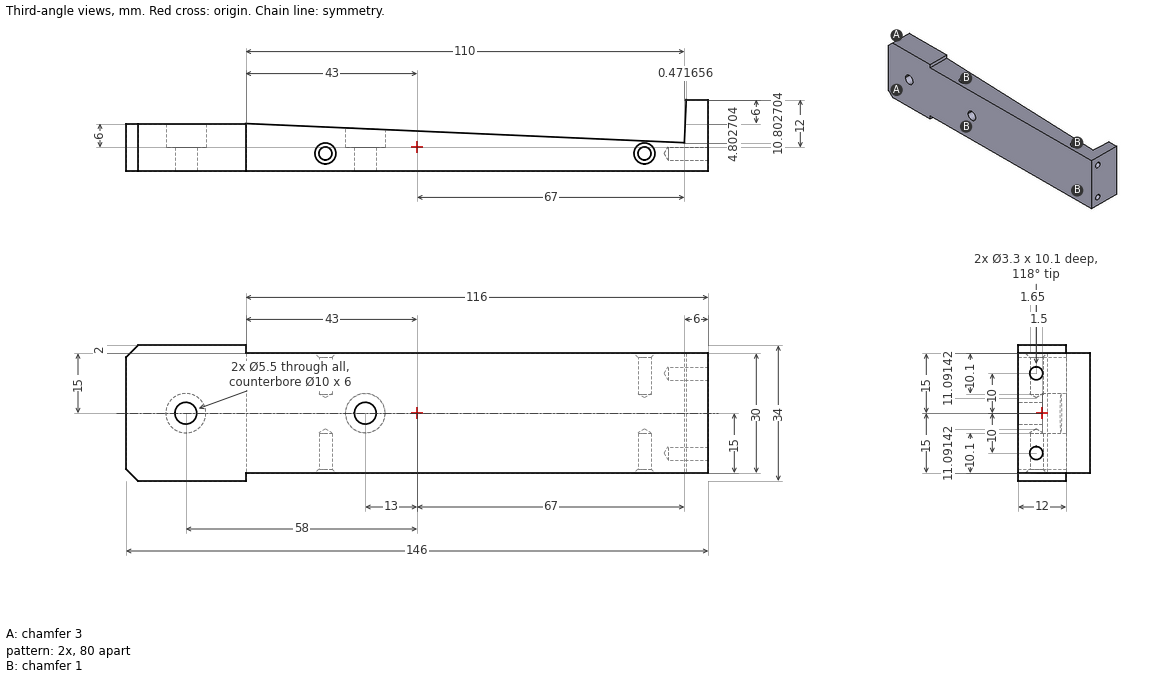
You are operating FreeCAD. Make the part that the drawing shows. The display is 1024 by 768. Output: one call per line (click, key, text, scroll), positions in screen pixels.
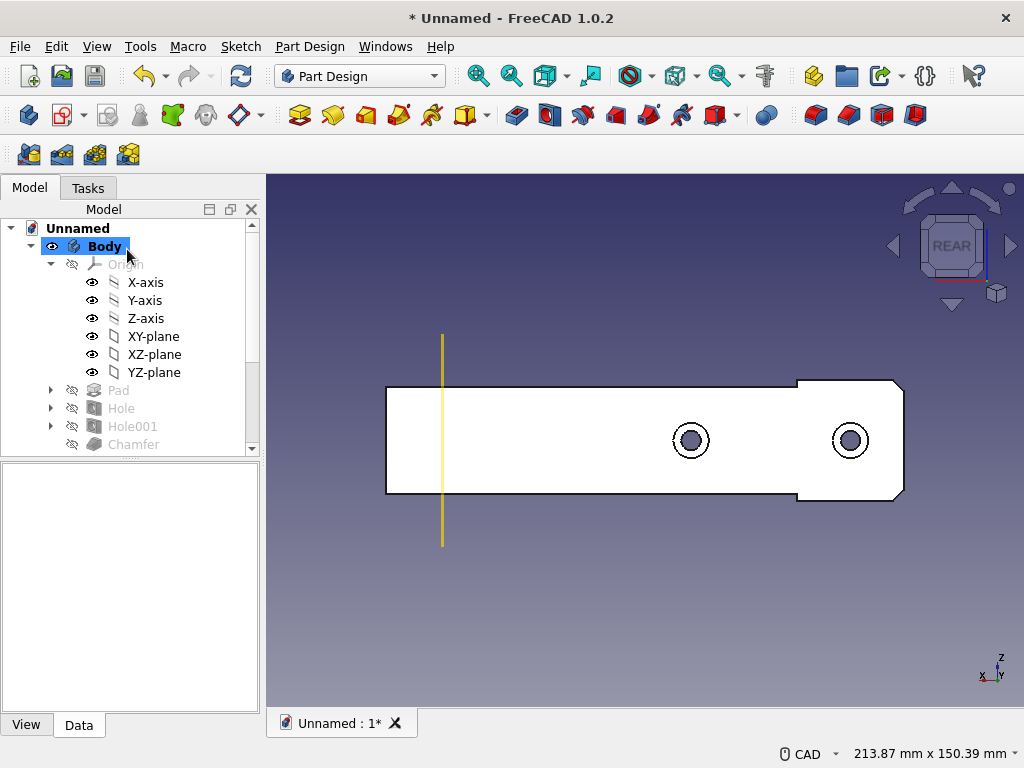
scroll(101, 332, down, 3)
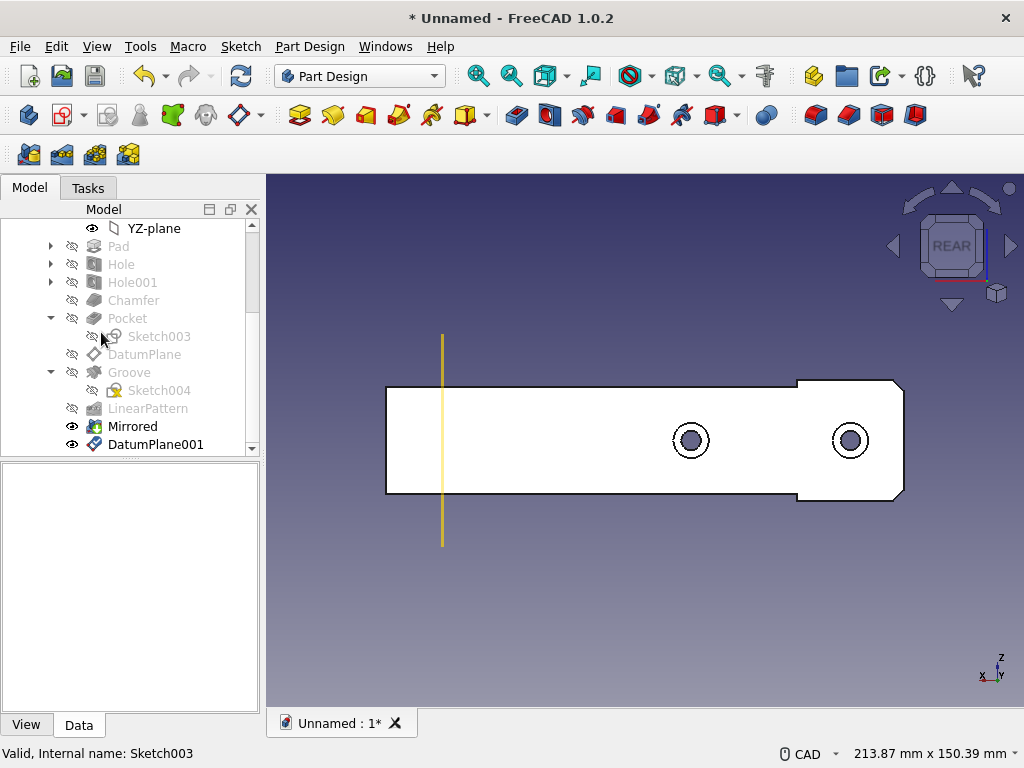
click(117, 444)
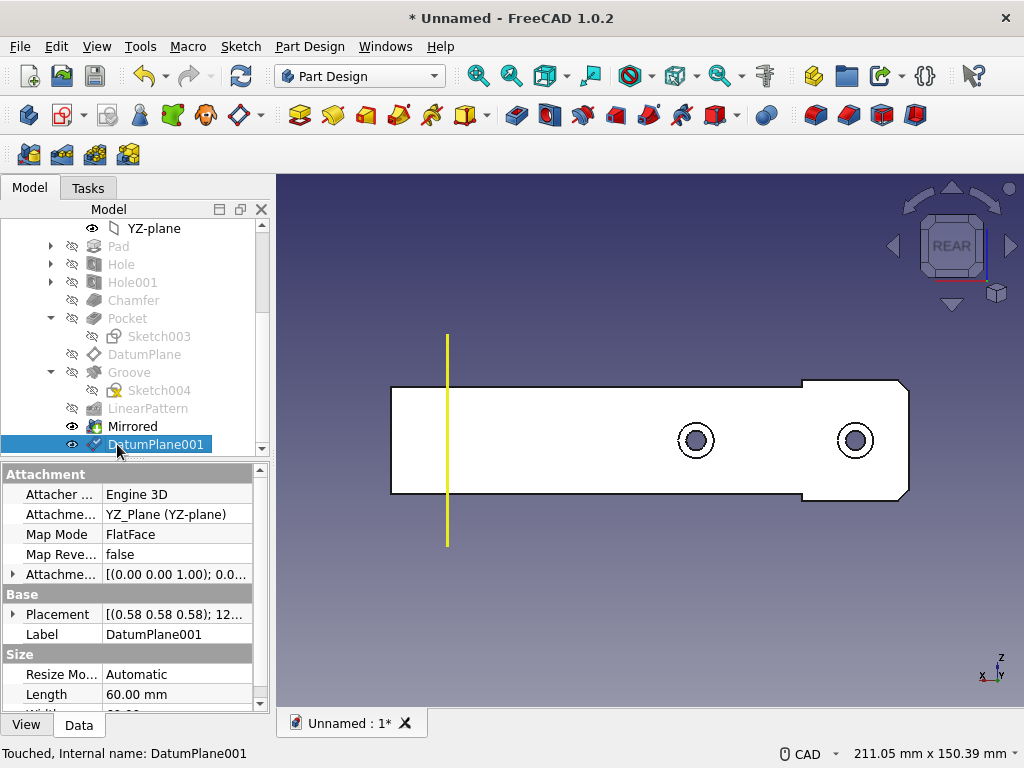
click(62, 116)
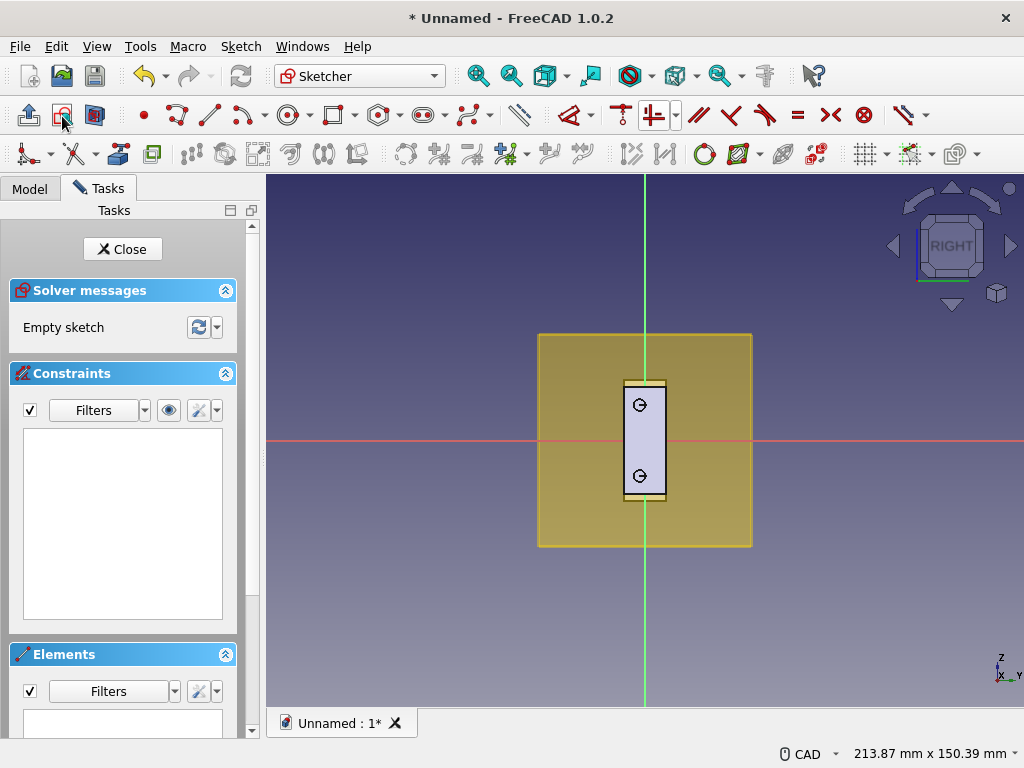
key(q)
key(s)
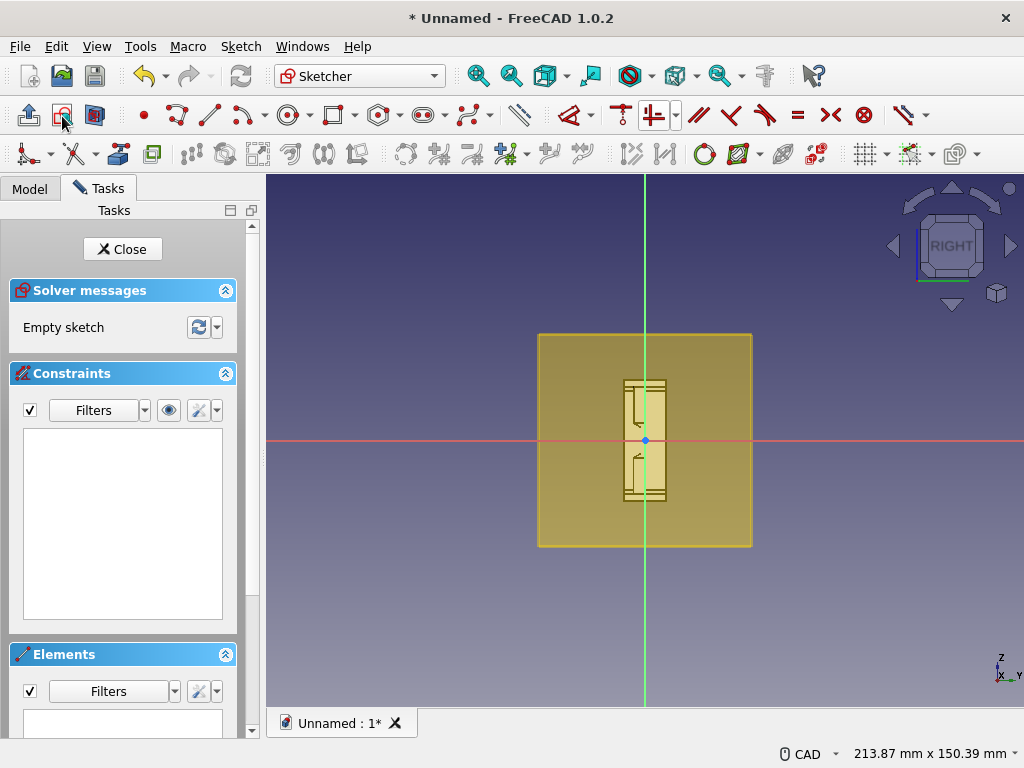
scroll(655, 484, up, 8)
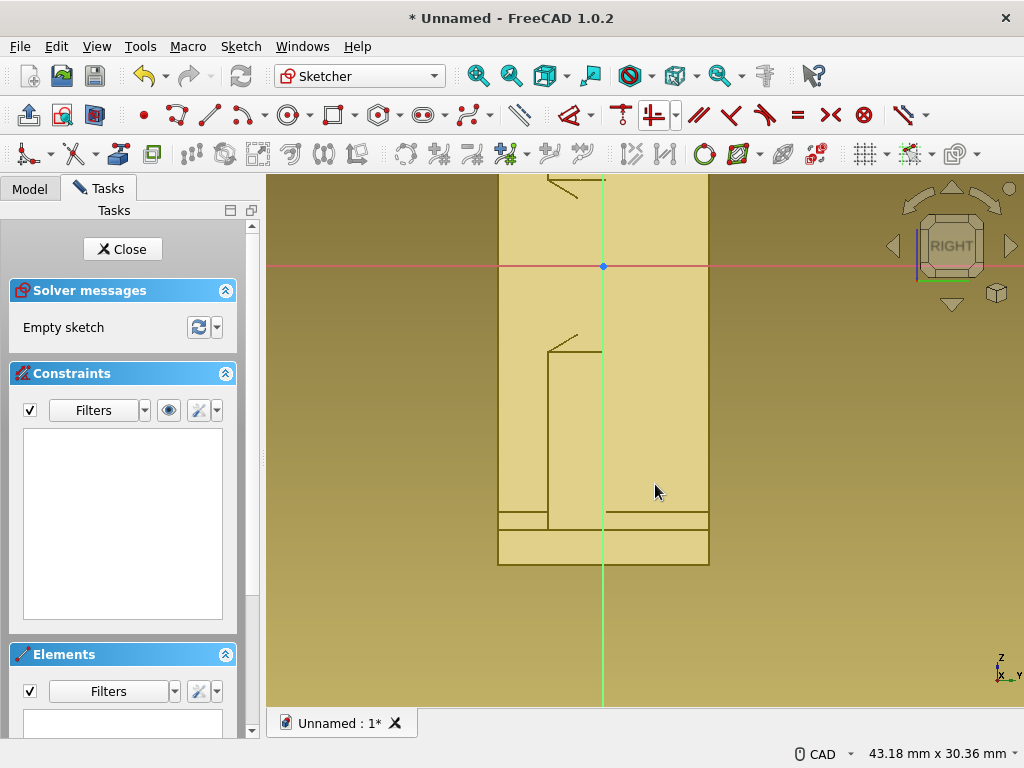
key(g)
key(m)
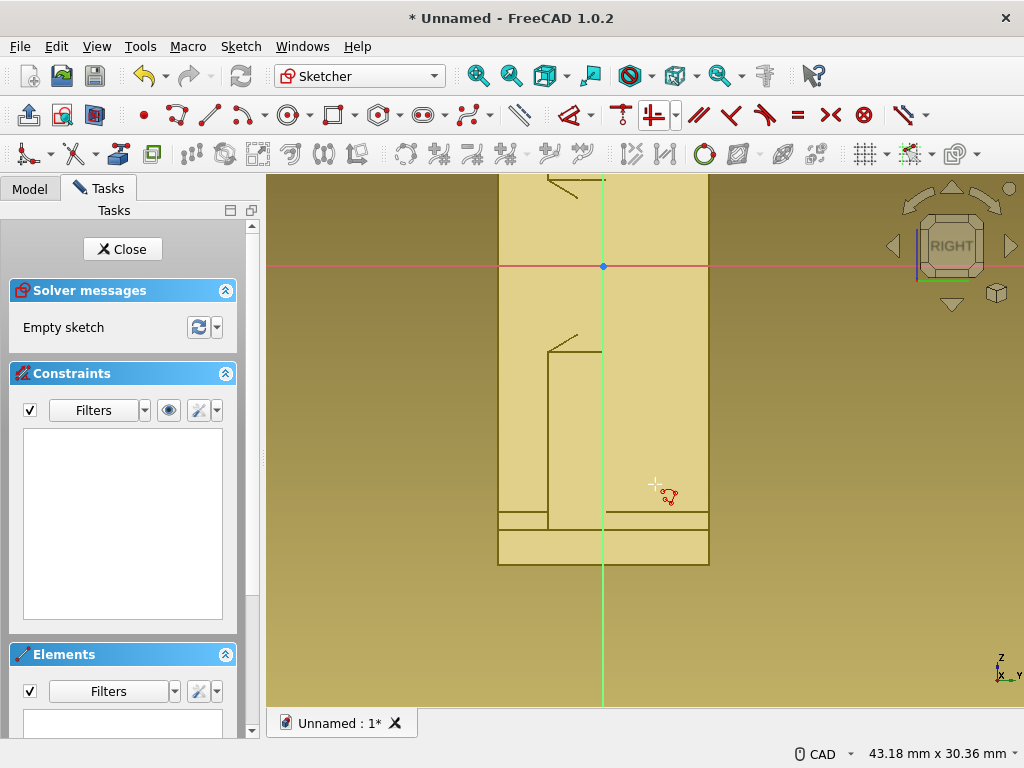
click(577, 335)
click(548, 352)
click(548, 530)
click(577, 530)
click(577, 336)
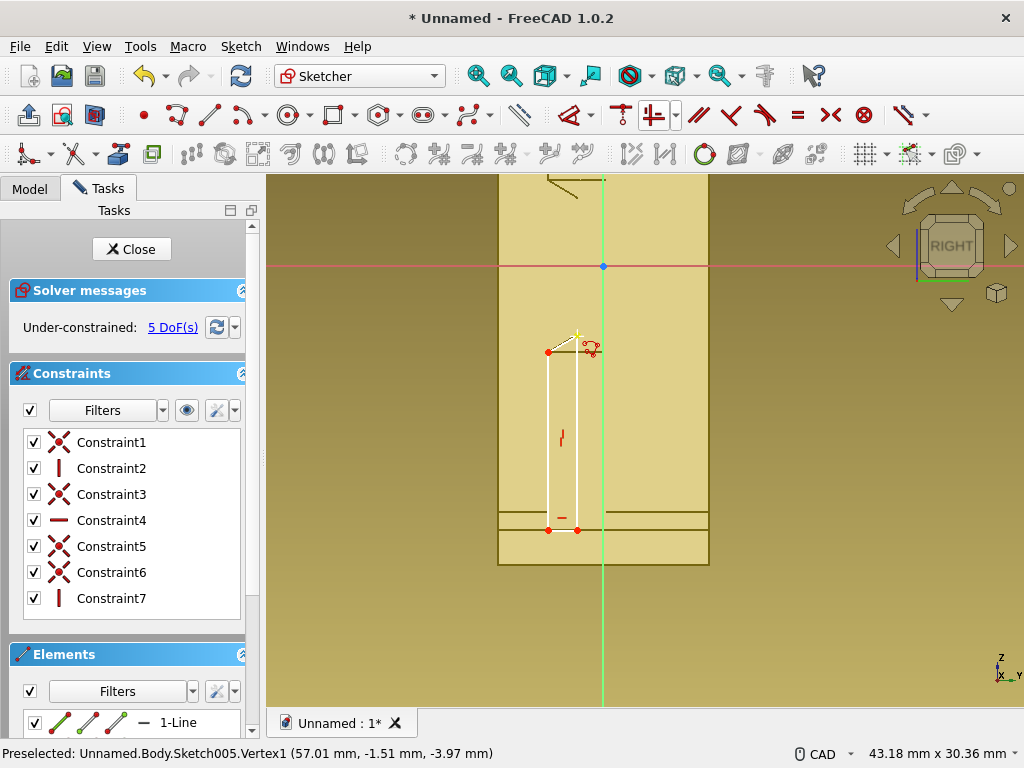
click(210, 116)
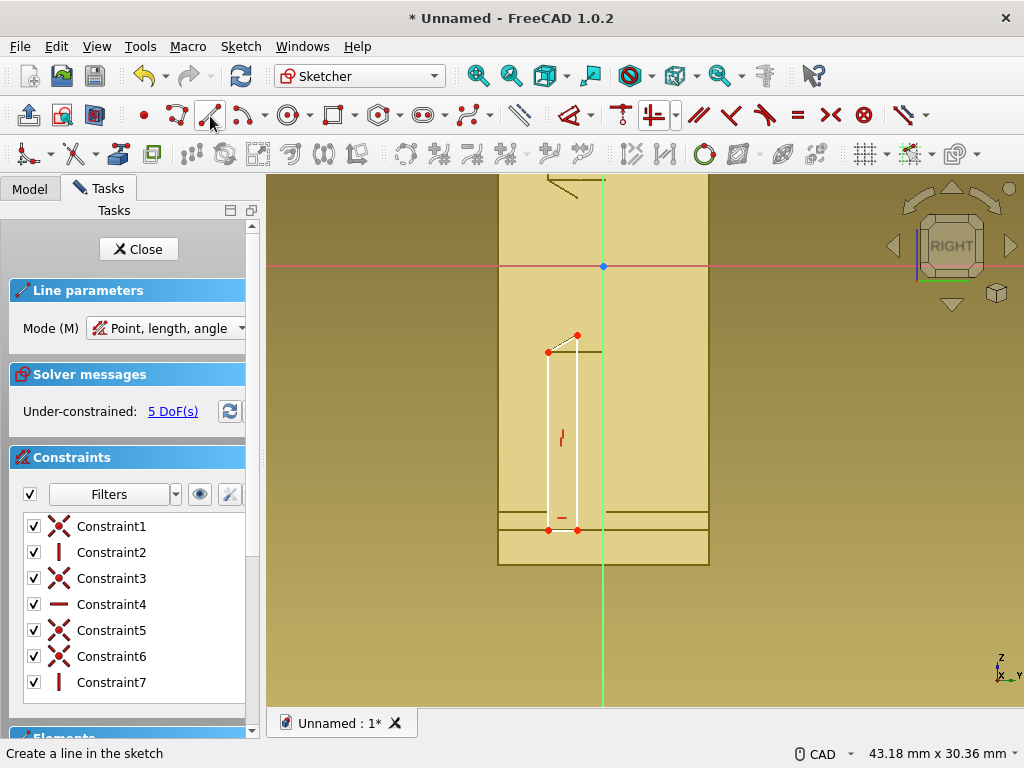
click(577, 549)
click(577, 607)
key(Escape)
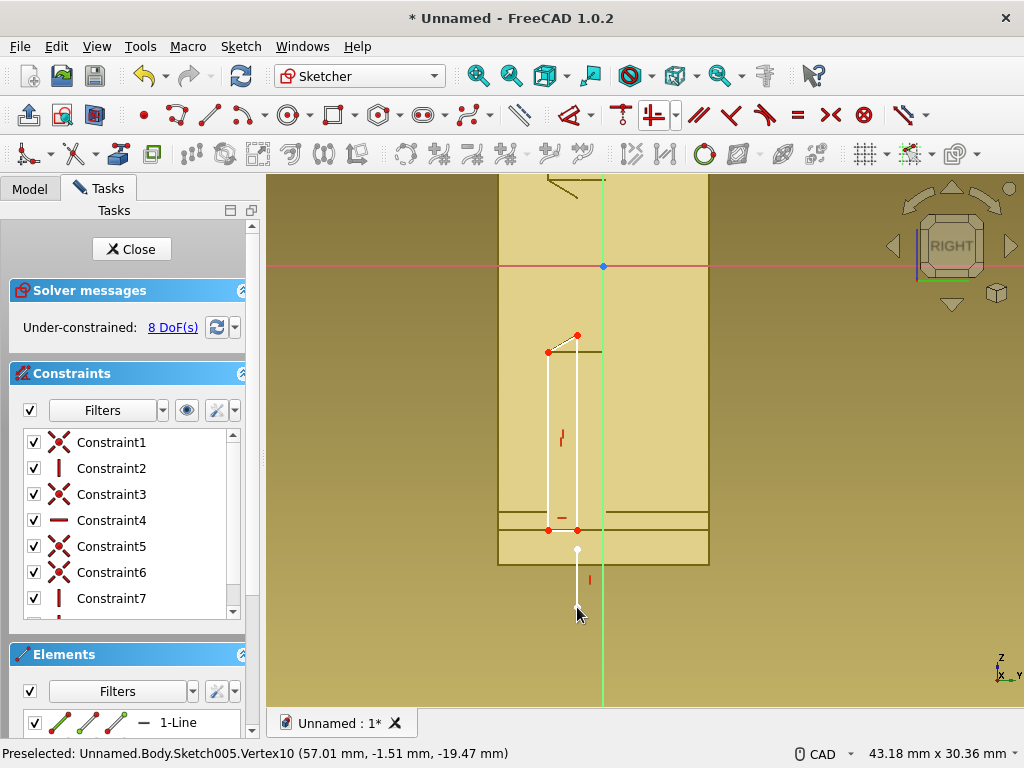
click(577, 567)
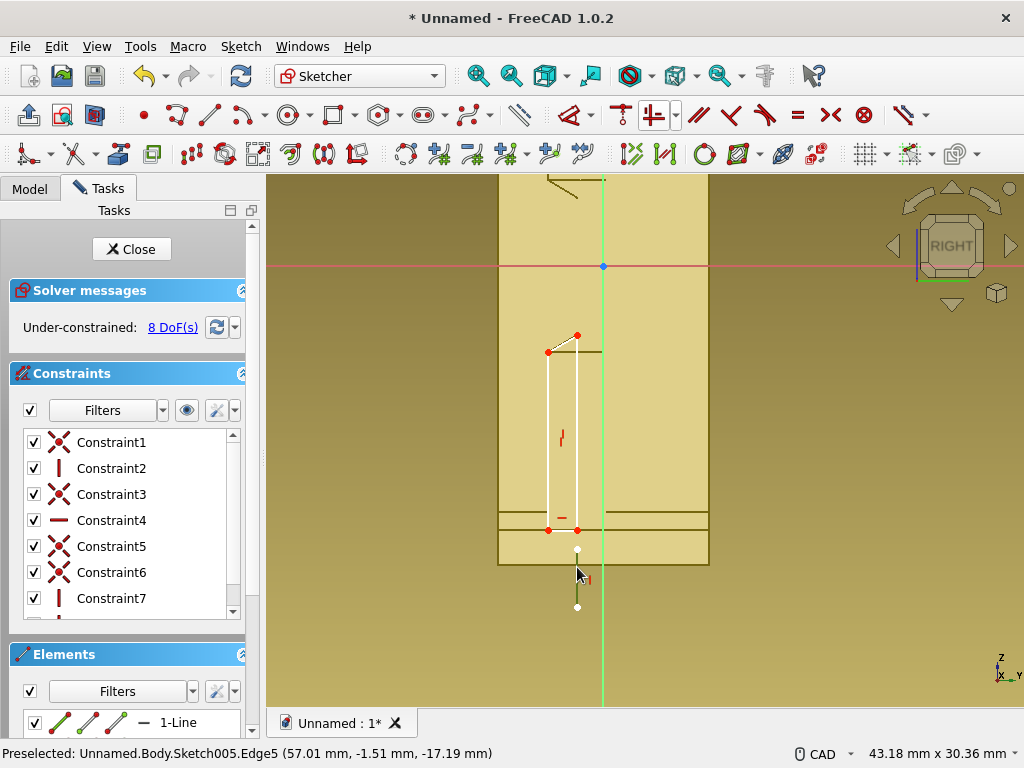
key(g)
key(n)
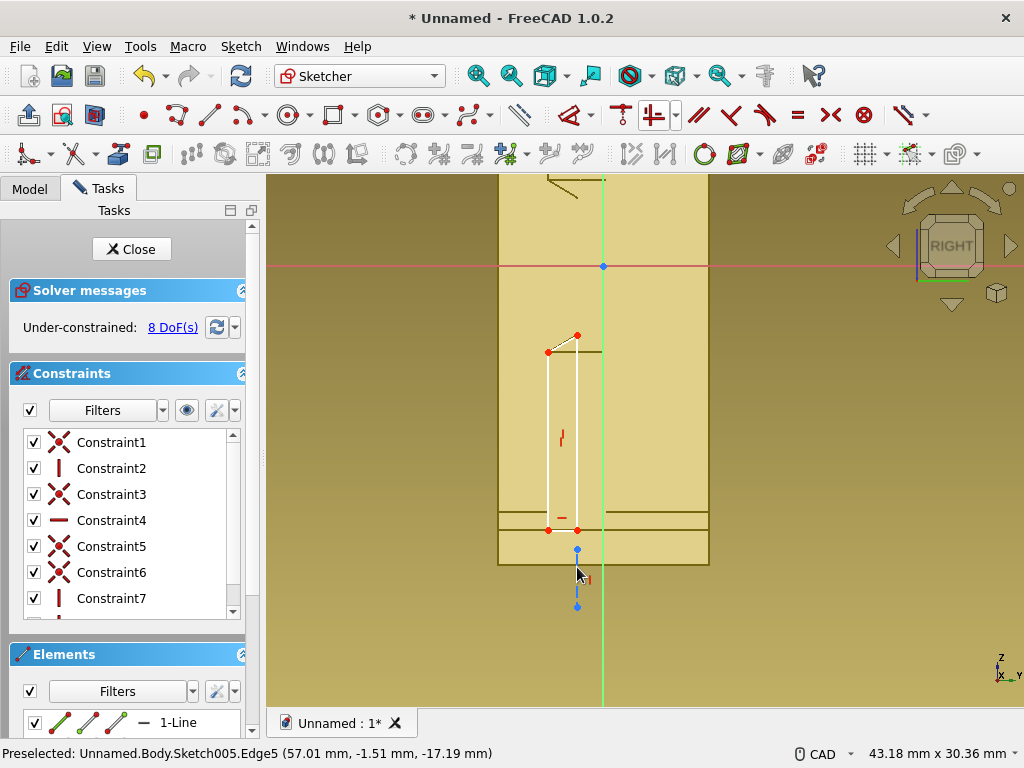
key(d)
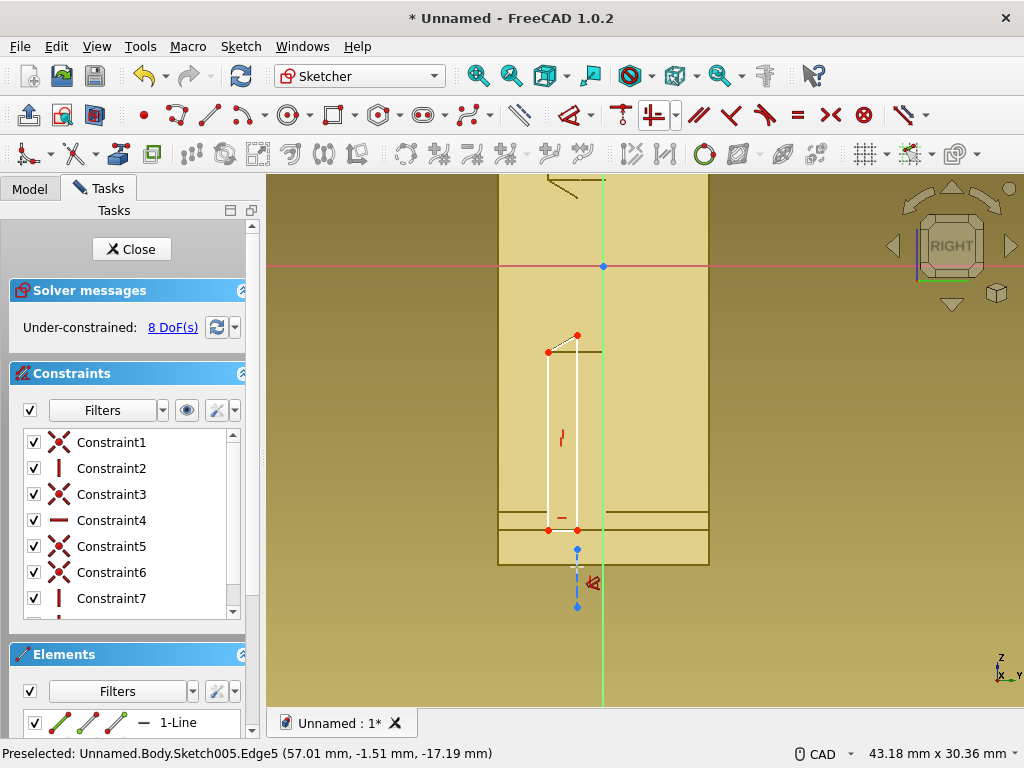
click(548, 531)
click(514, 399)